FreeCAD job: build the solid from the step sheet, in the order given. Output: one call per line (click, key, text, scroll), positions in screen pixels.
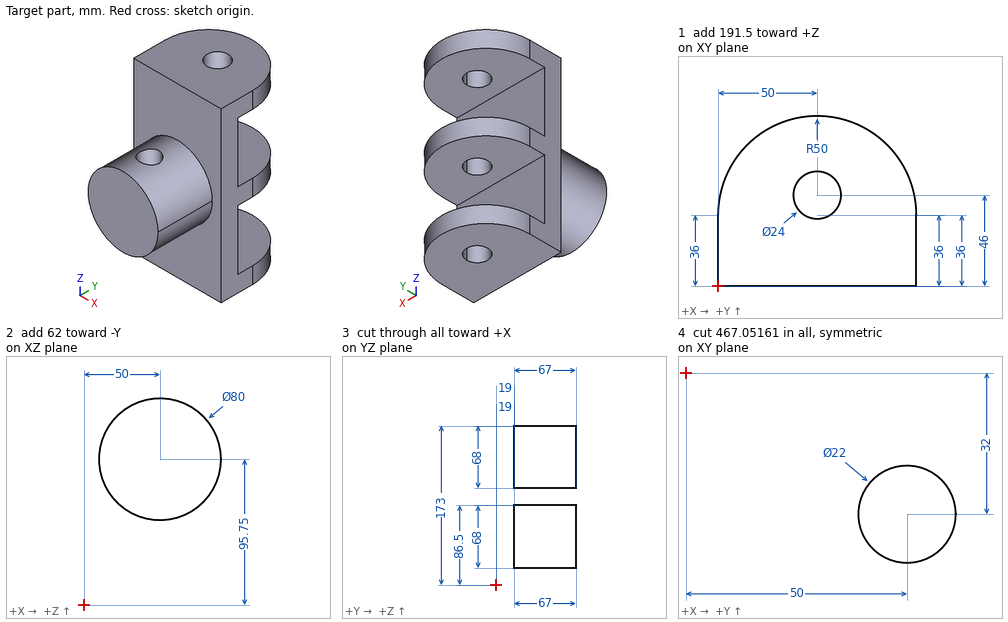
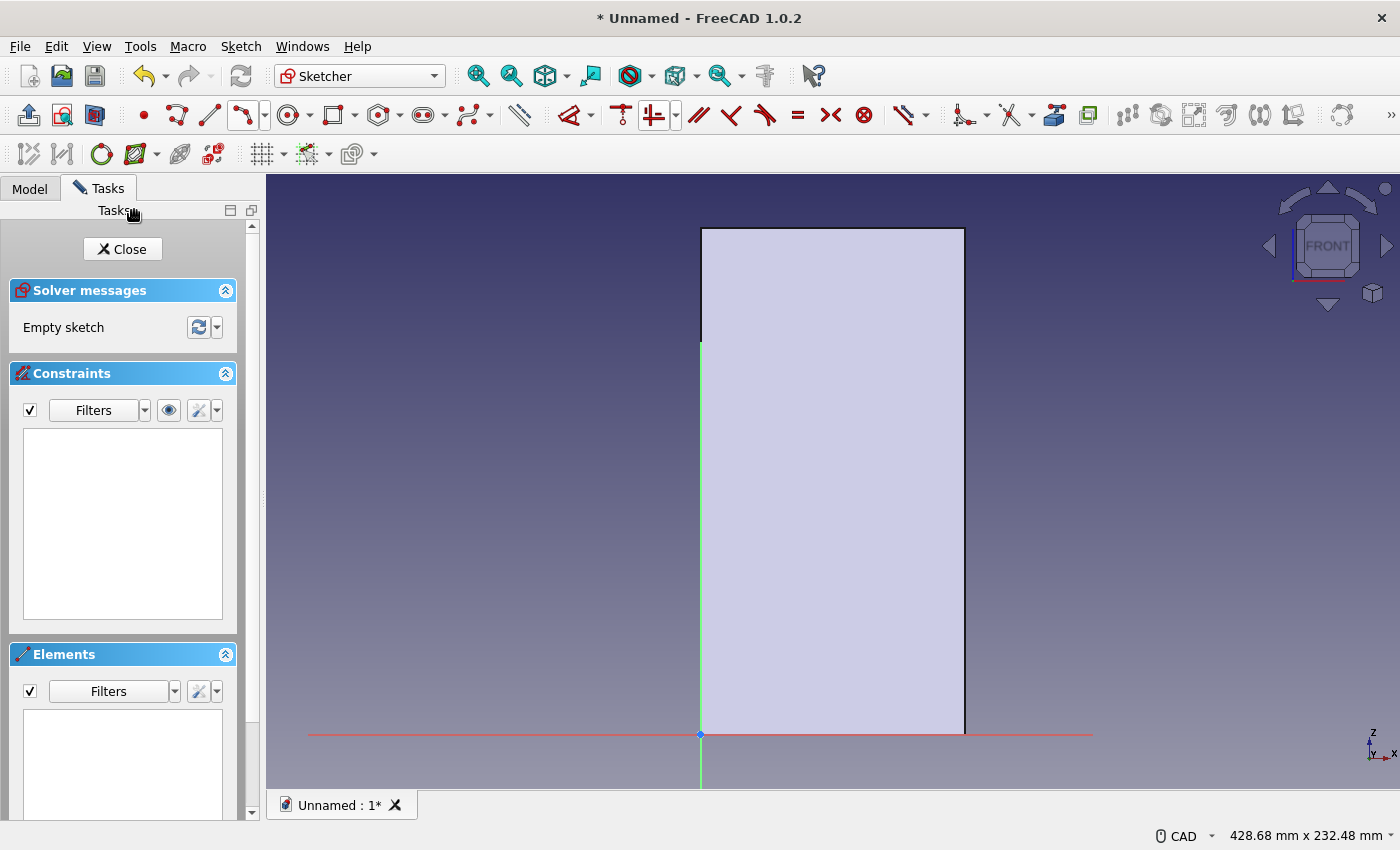
click(288, 116)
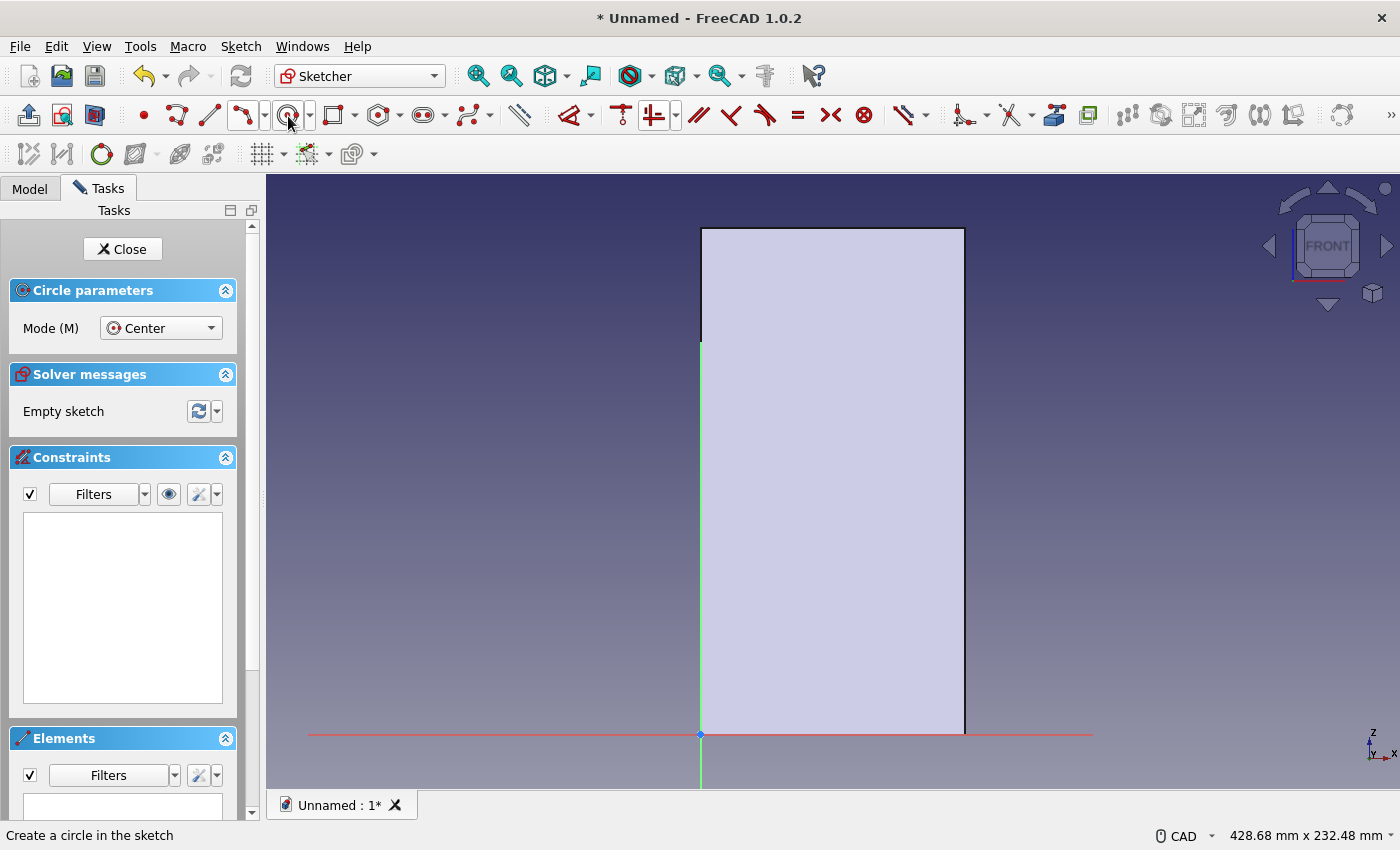
click(833, 482)
click(908, 407)
key(Escape)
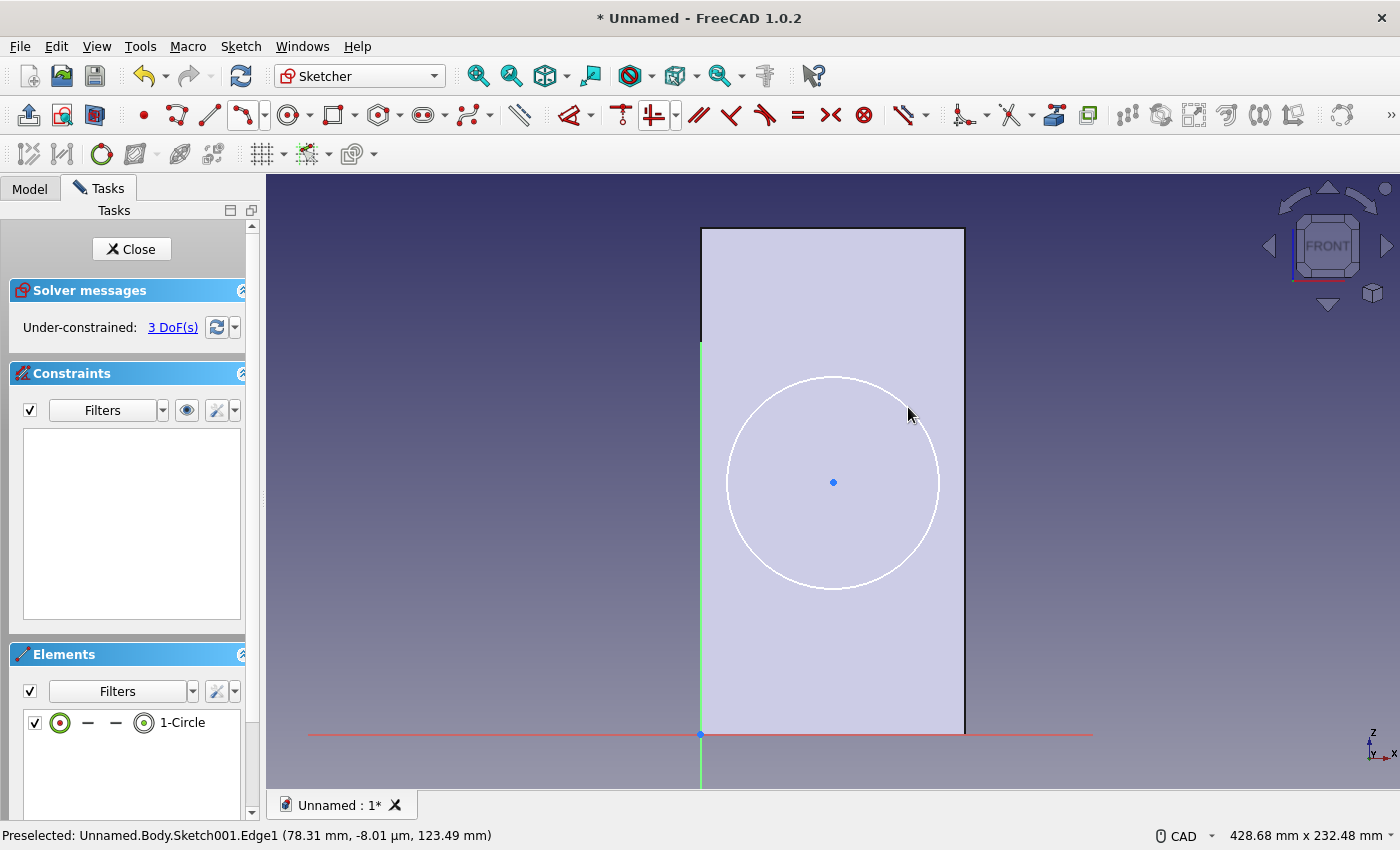
click(568, 116)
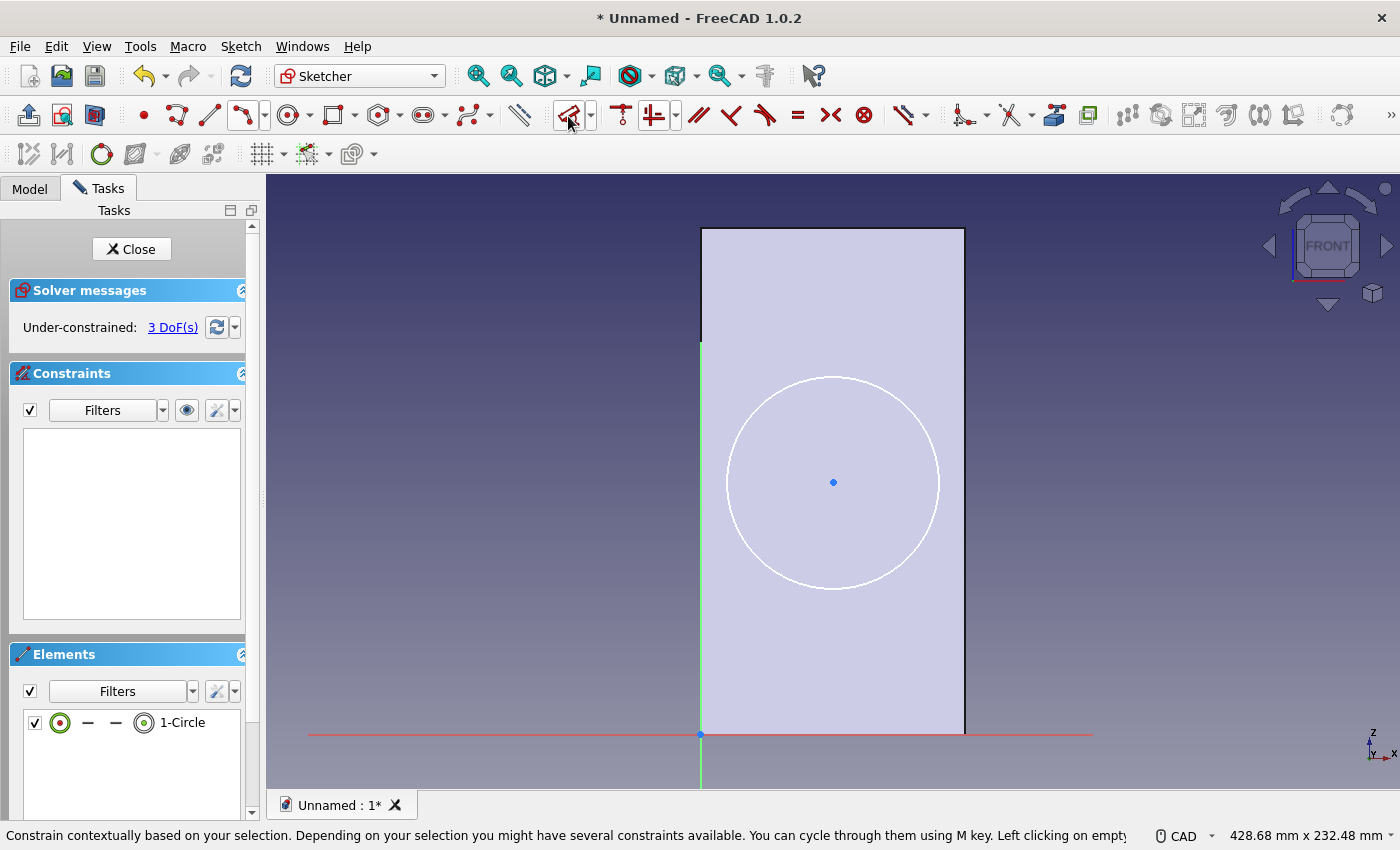
click(908, 408)
click(931, 385)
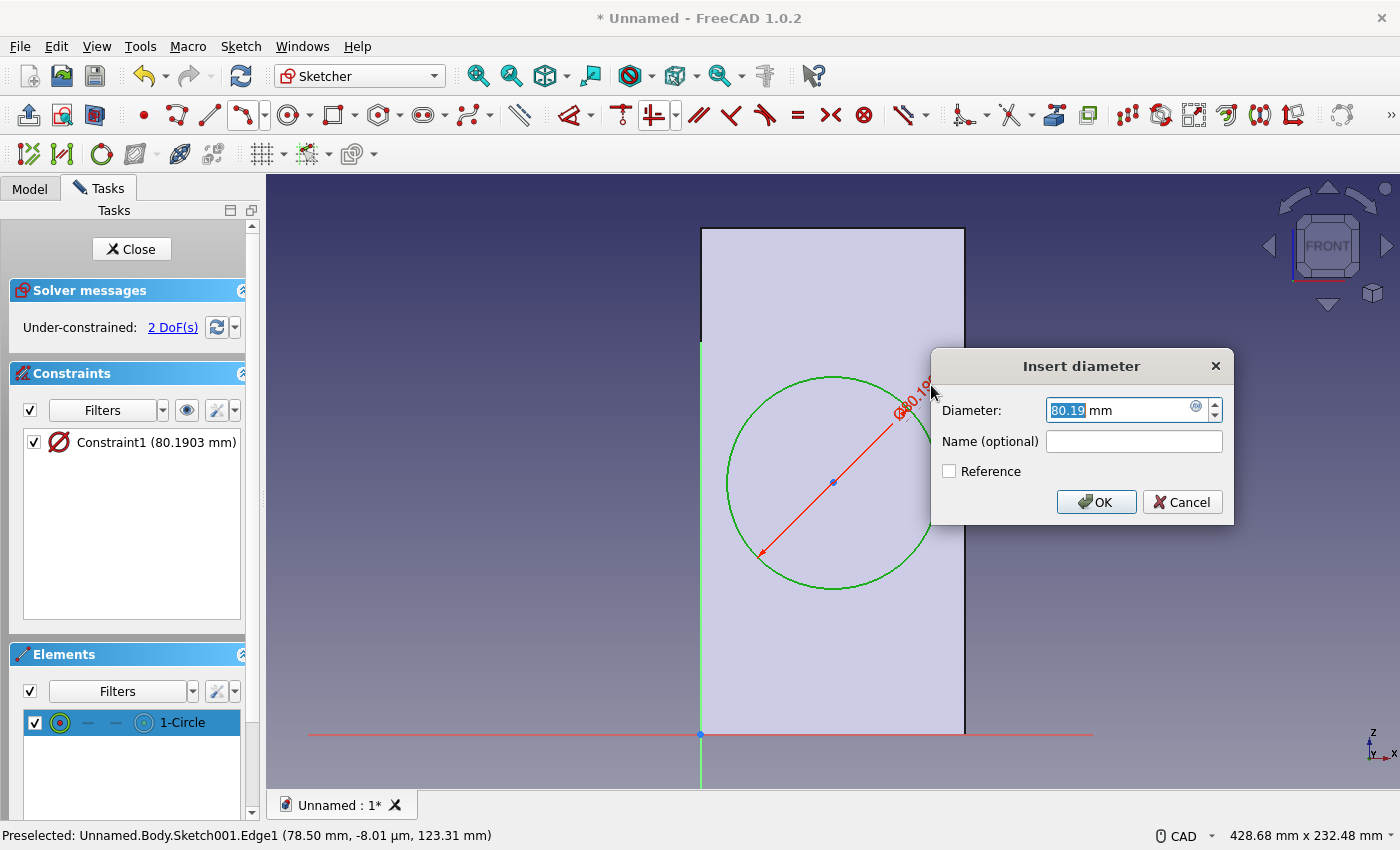
text(80)
key(Return)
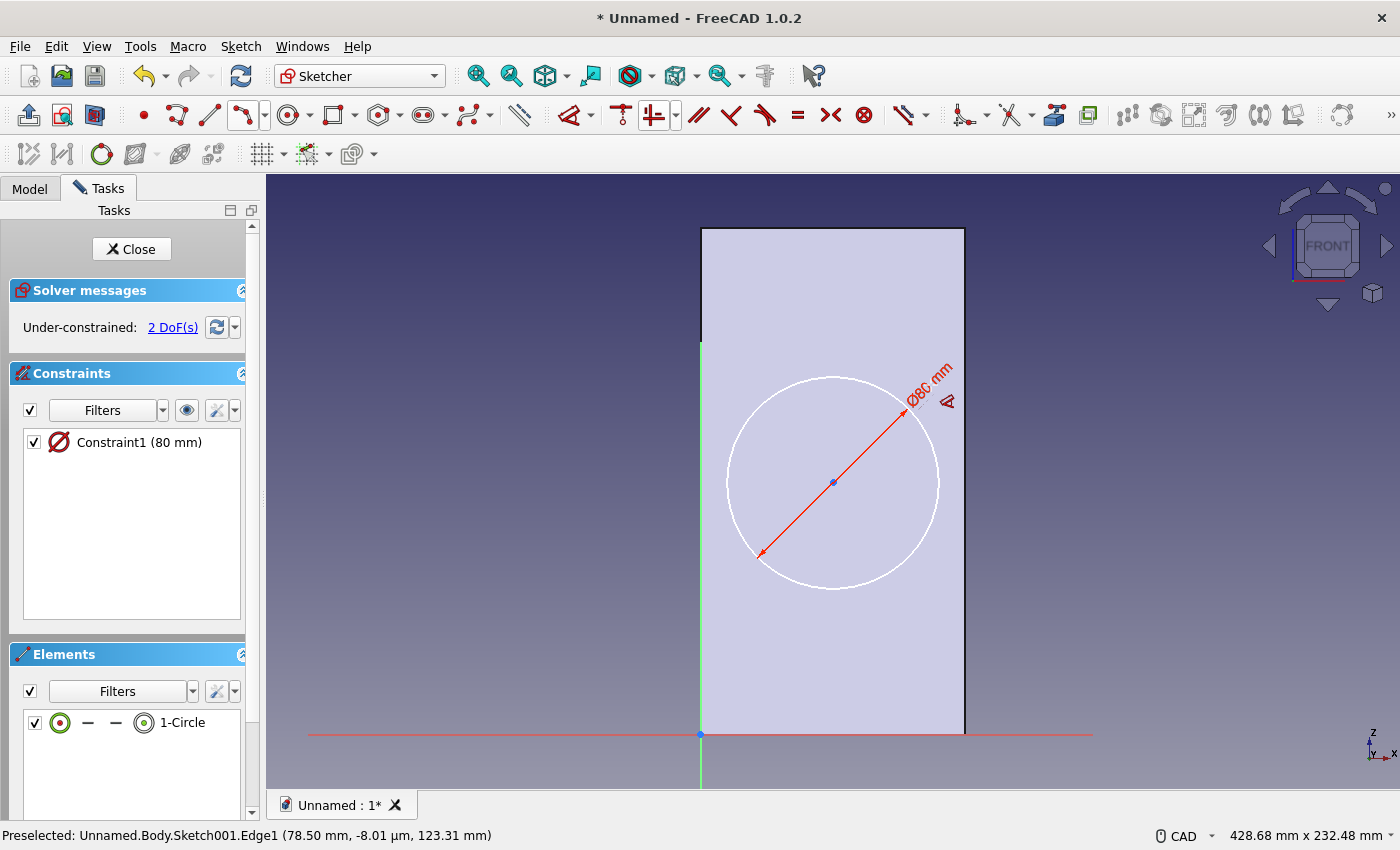
click(833, 483)
click(767, 449)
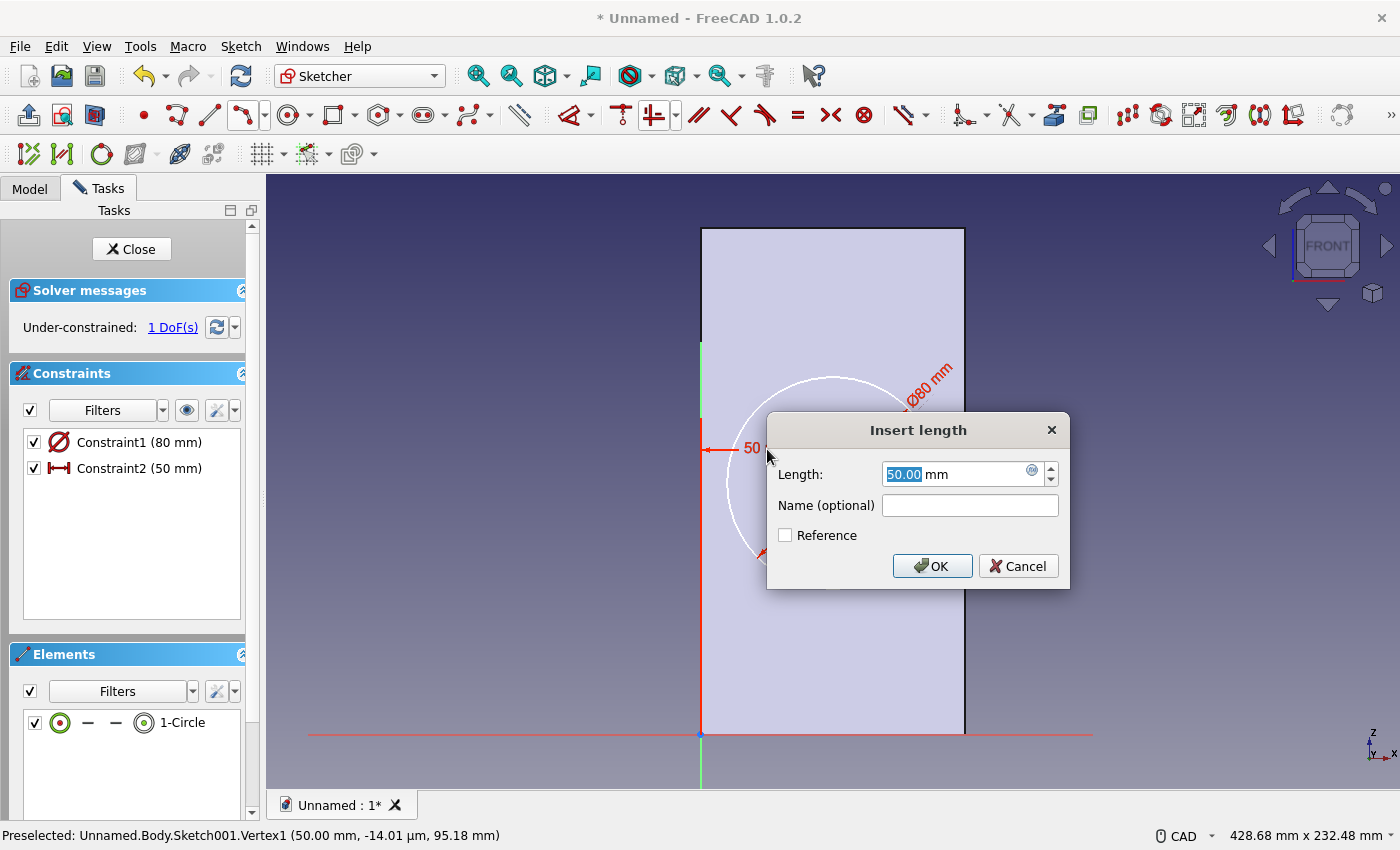
text(50)
key(Return)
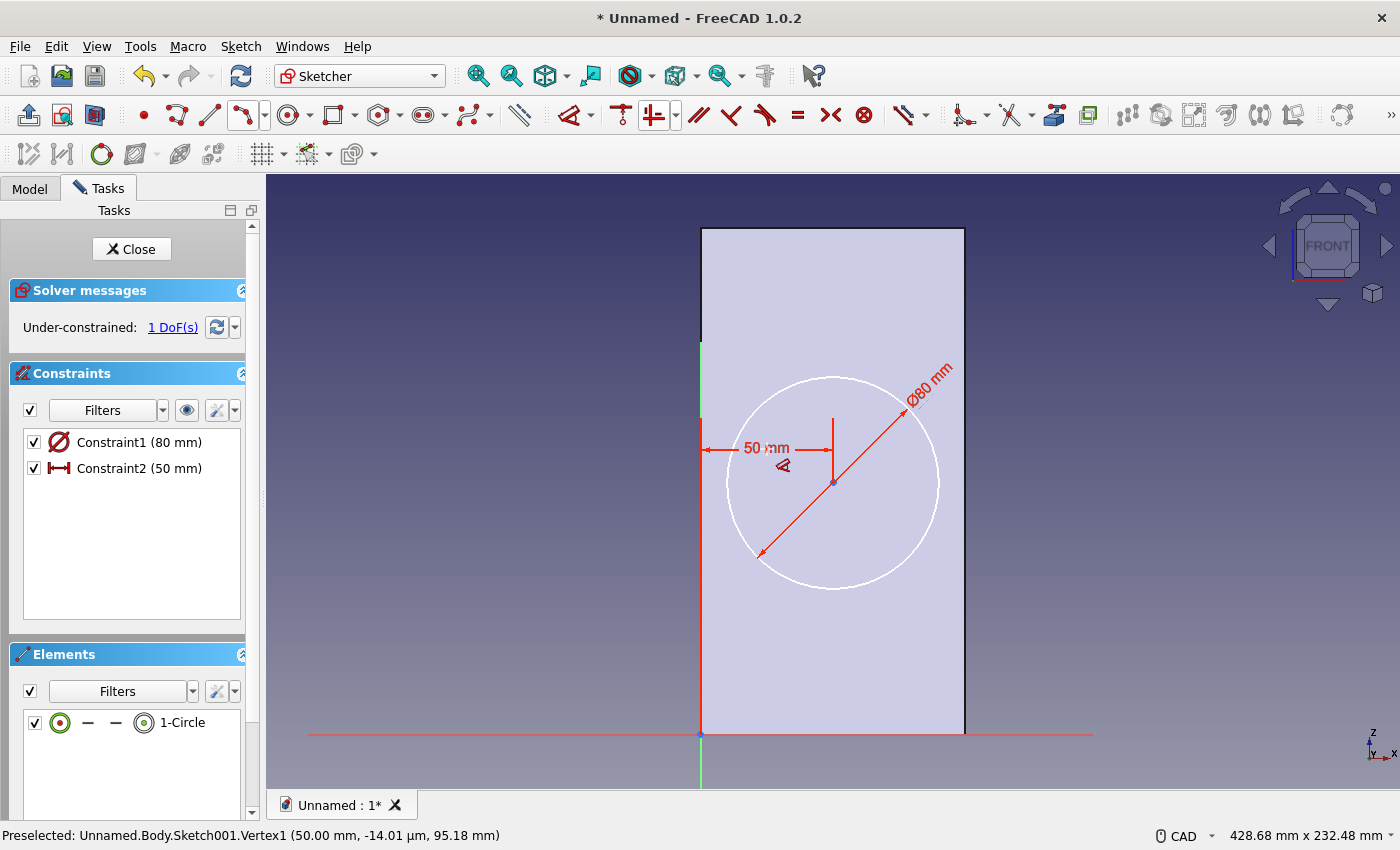
click(833, 483)
click(667, 609)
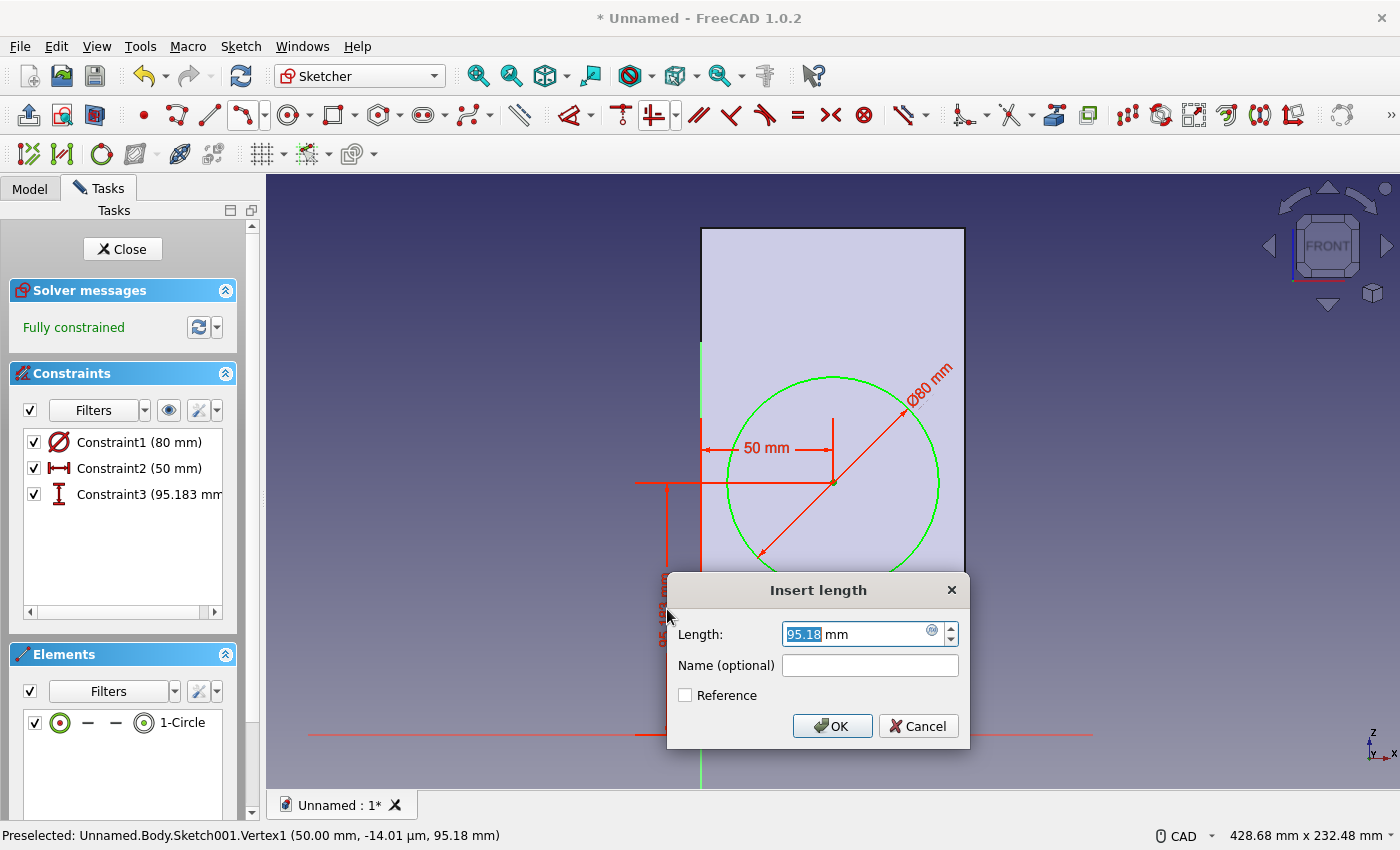
text(95.75)
key(Return)
key(Escape)